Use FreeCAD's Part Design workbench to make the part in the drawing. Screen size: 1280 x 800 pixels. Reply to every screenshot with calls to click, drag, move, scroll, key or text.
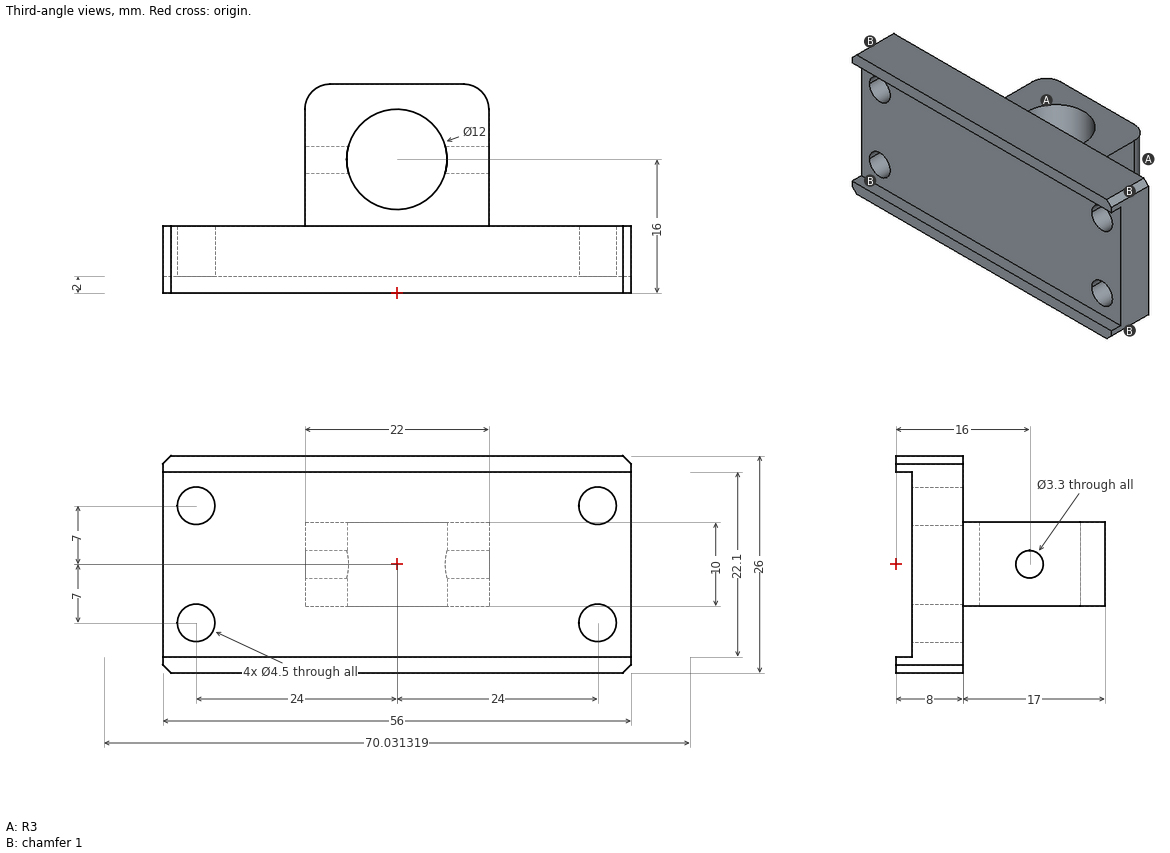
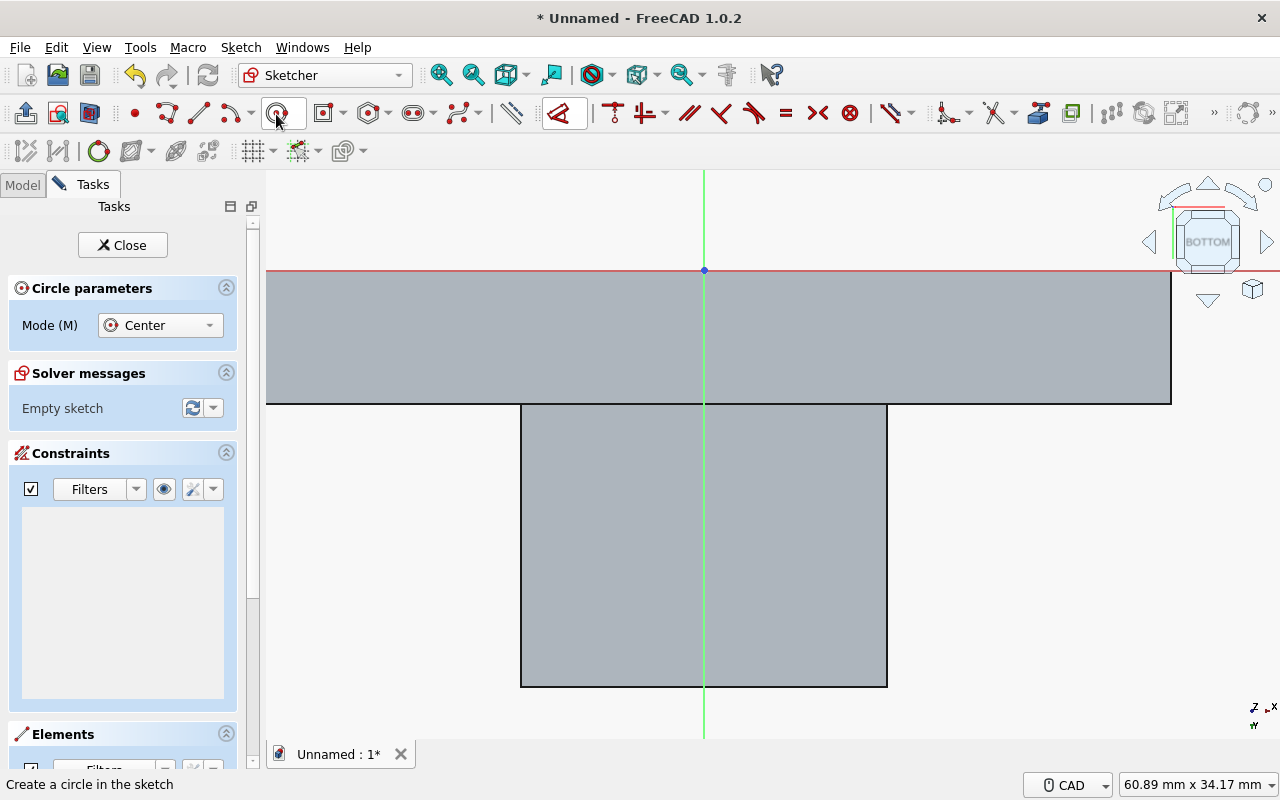
click(704, 537)
move(775, 467)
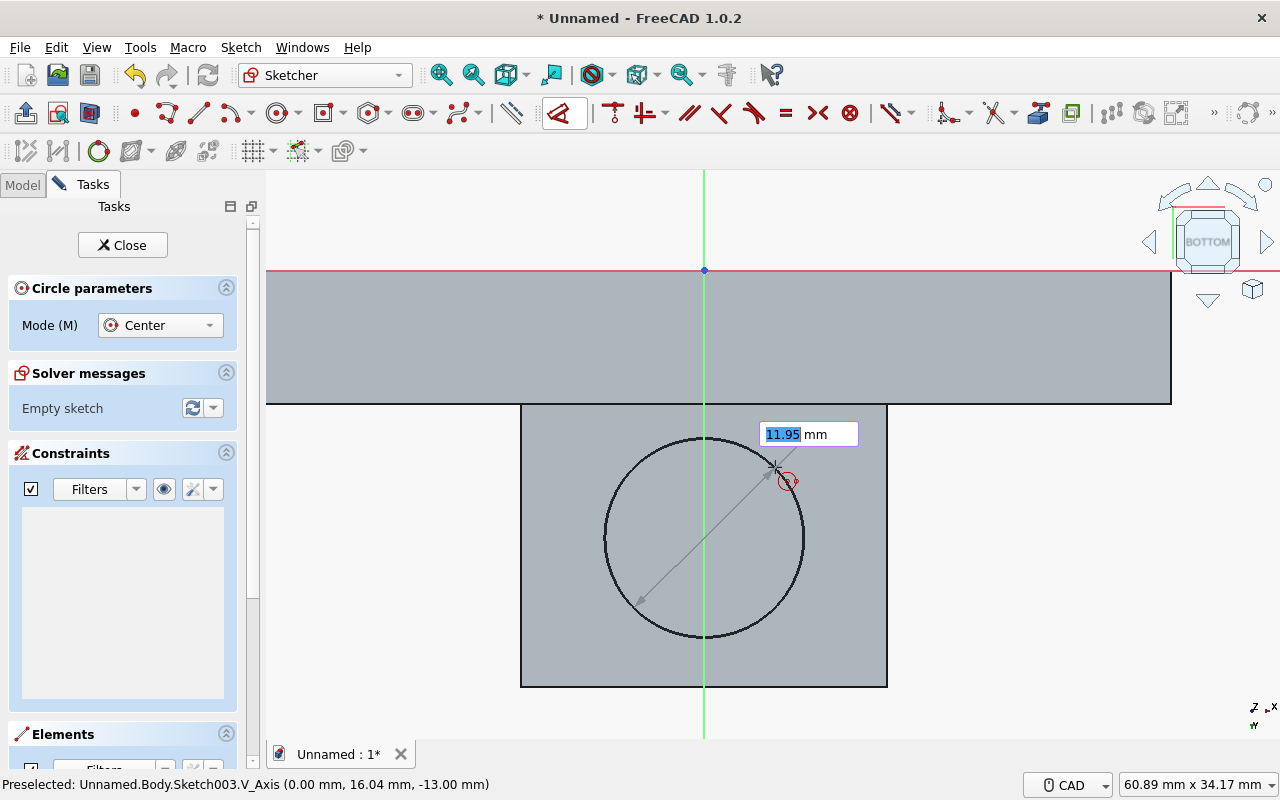
text(12)
key(Return)
key(Escape)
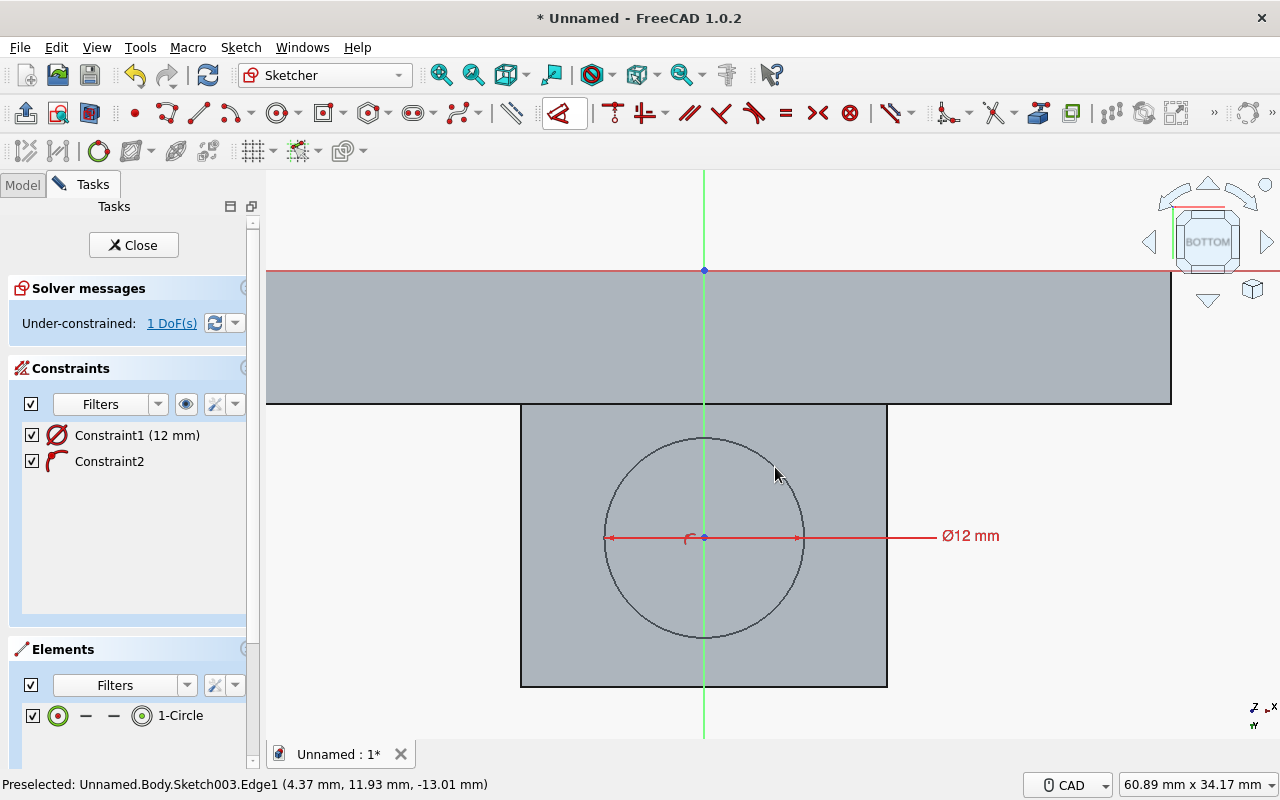
click(558, 114)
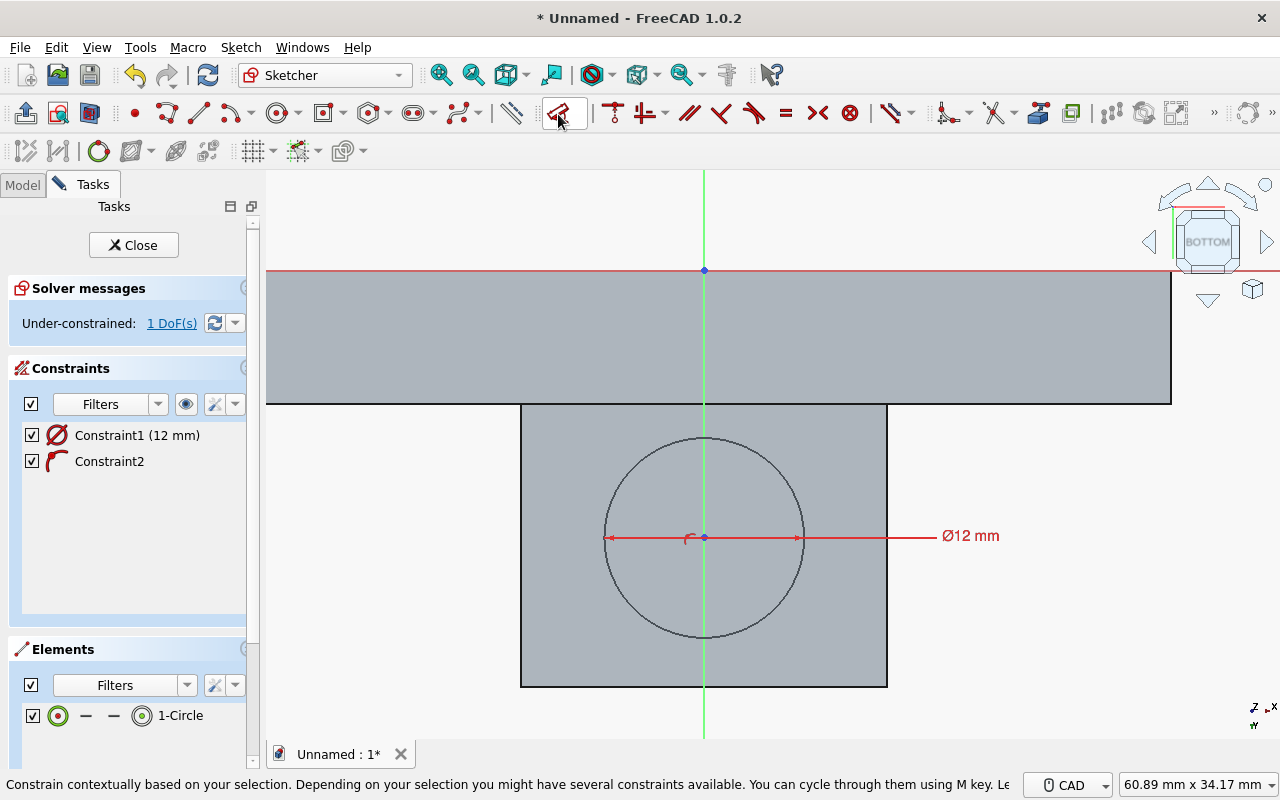
click(704, 538)
click(738, 404)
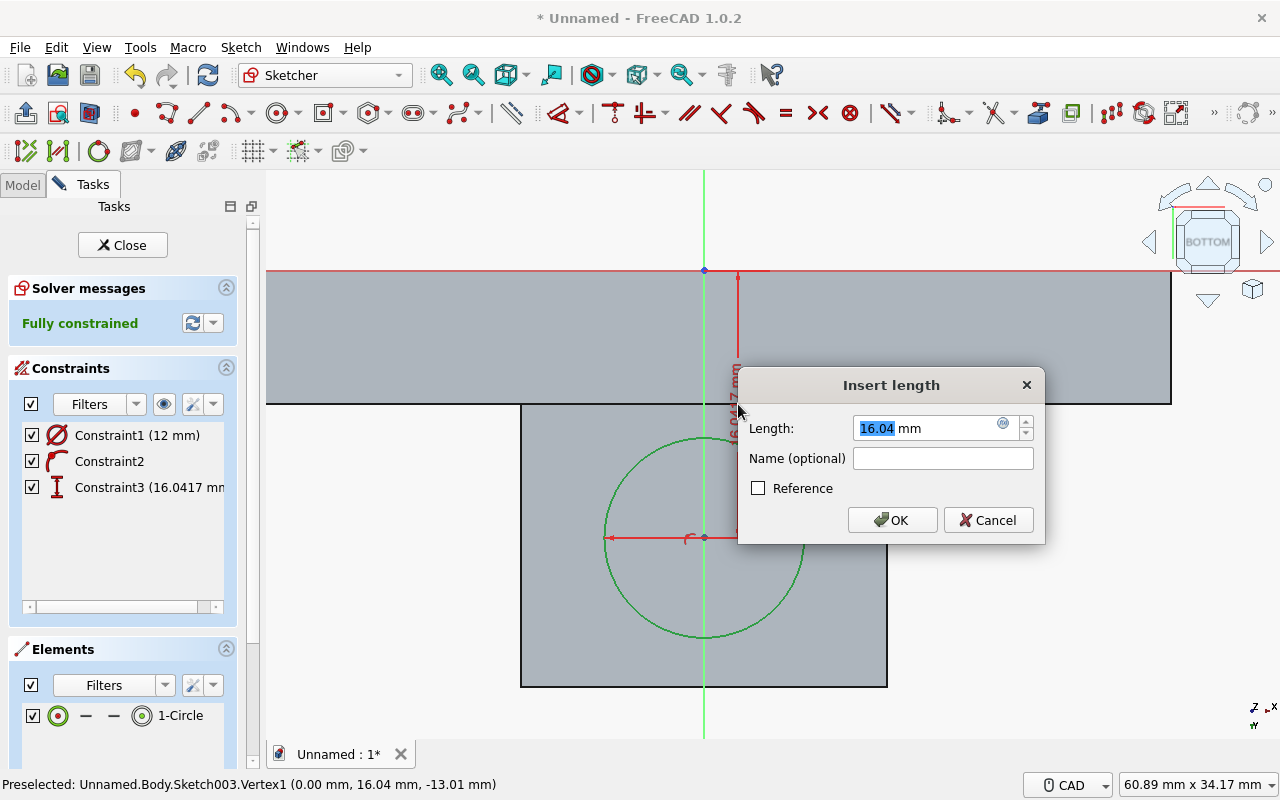
text(16)
key(Return)
key(Escape)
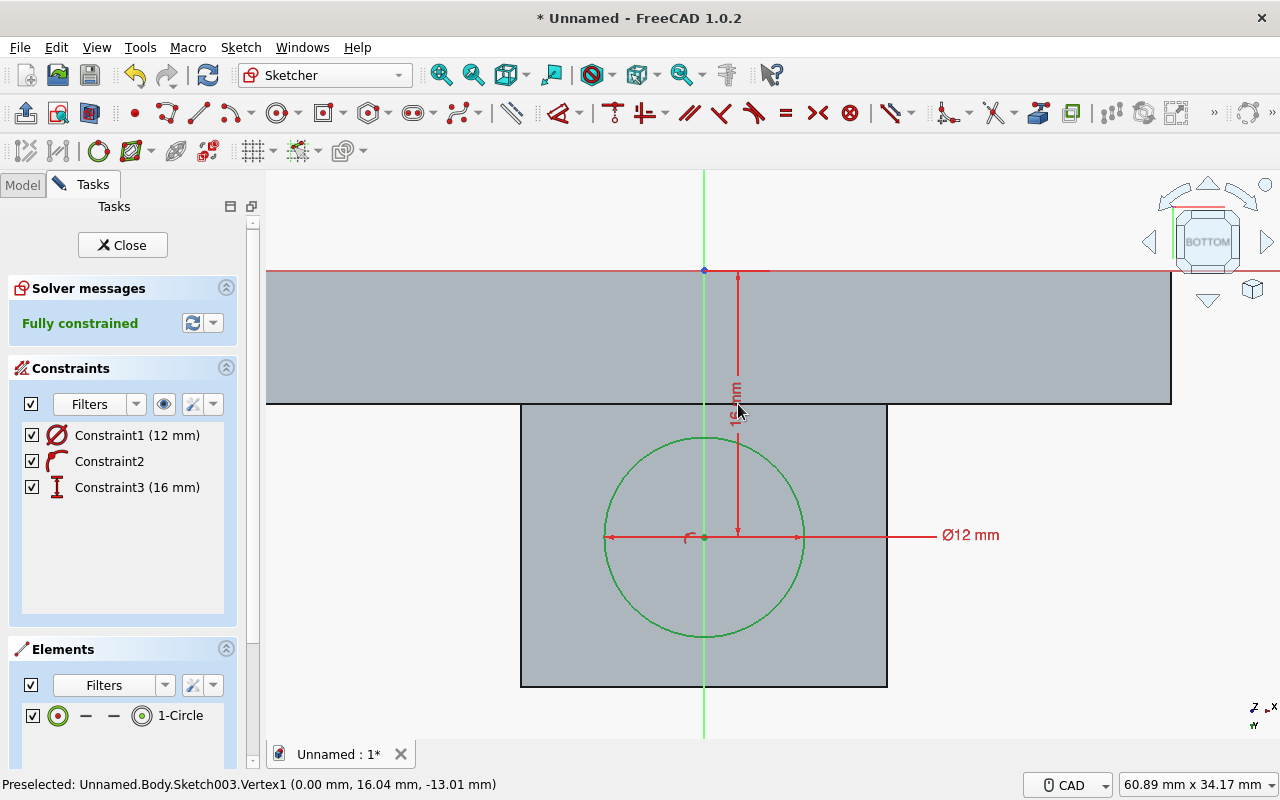
click(123, 245)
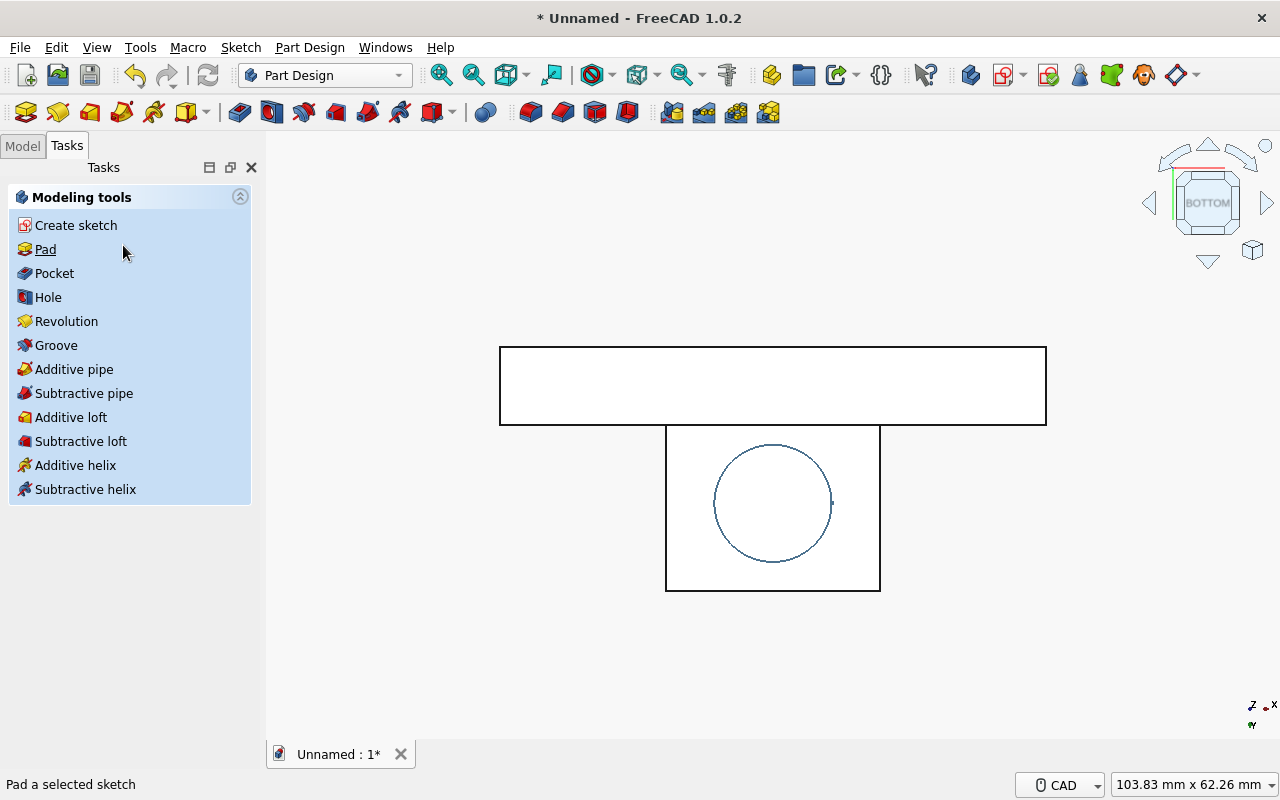
click(240, 112)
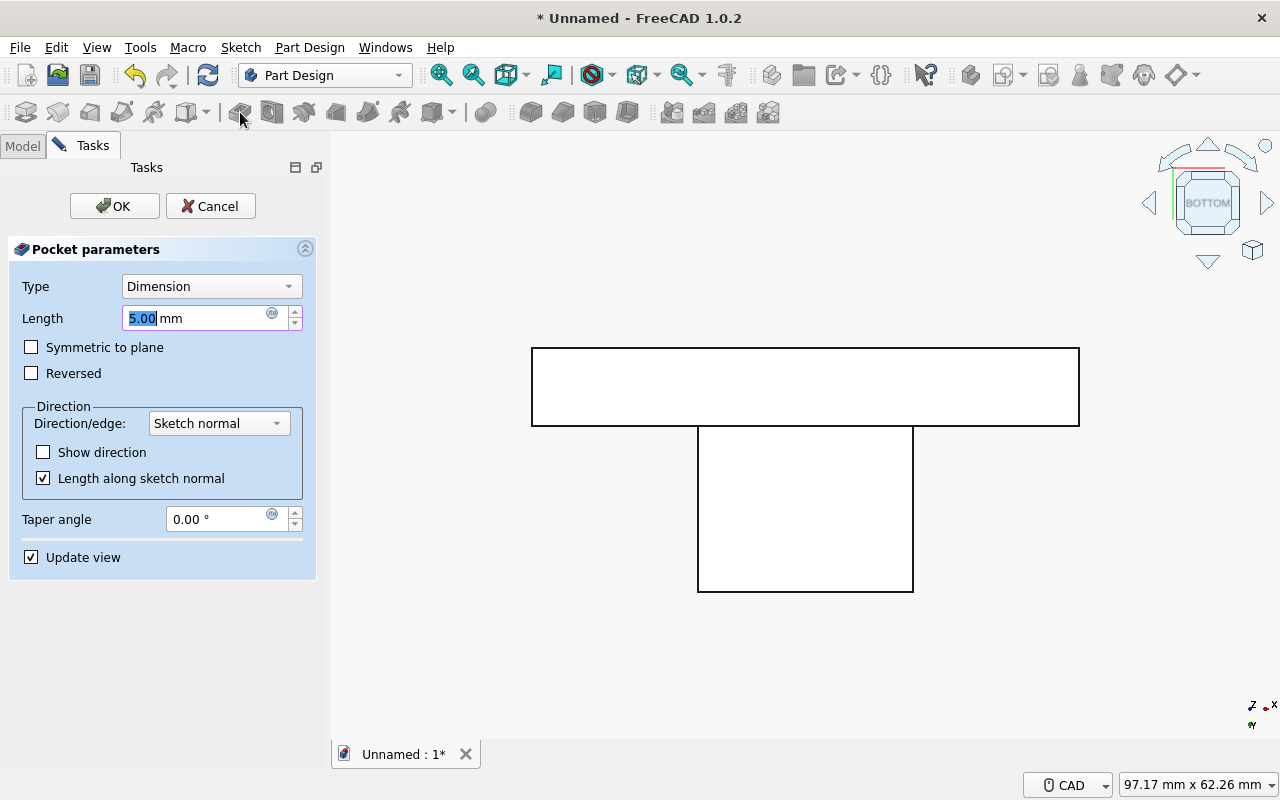
click(212, 286)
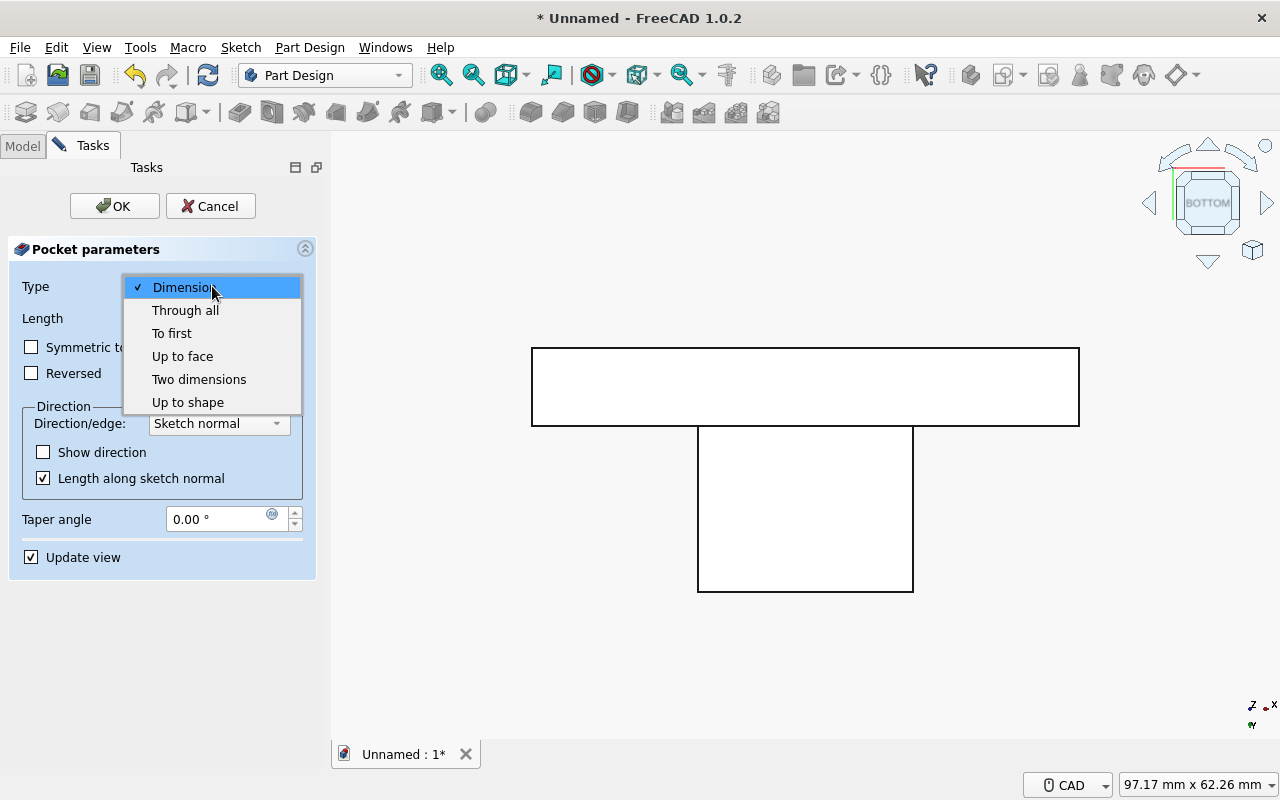
click(212, 310)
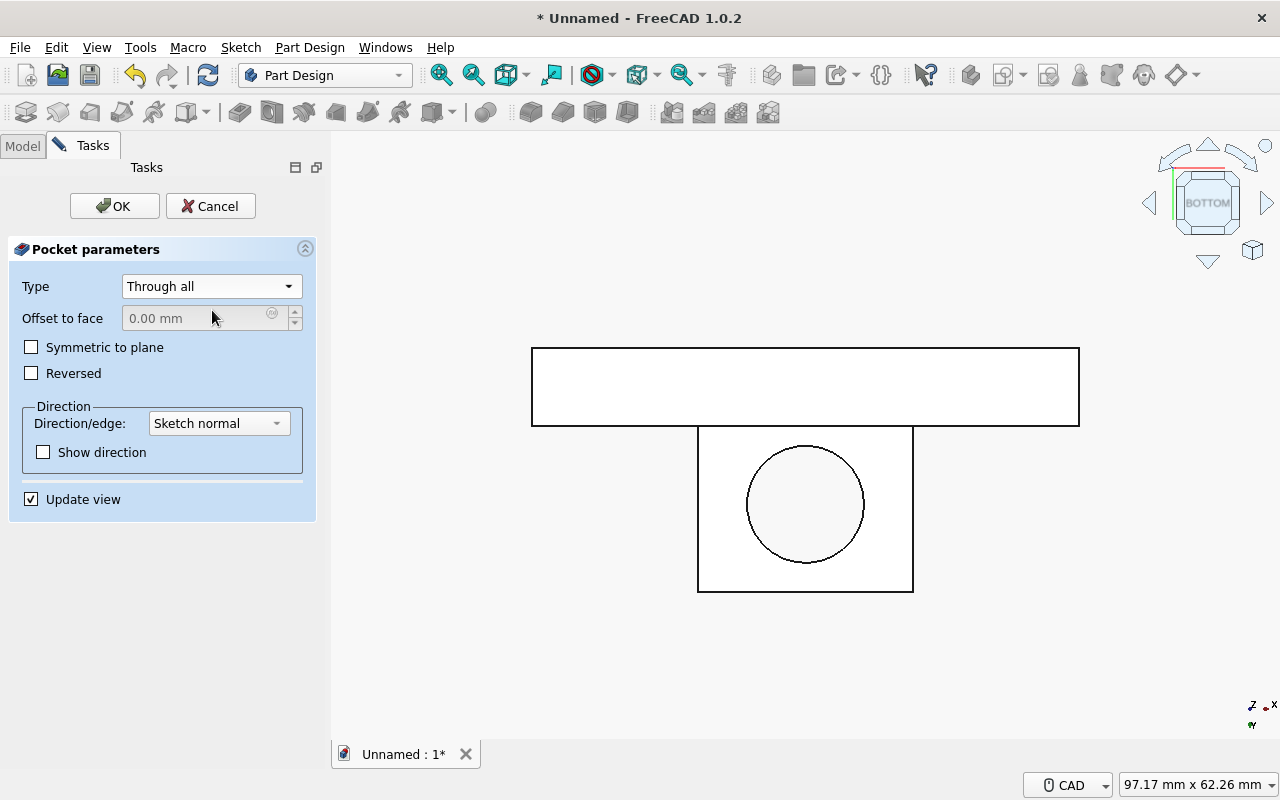
click(115, 206)